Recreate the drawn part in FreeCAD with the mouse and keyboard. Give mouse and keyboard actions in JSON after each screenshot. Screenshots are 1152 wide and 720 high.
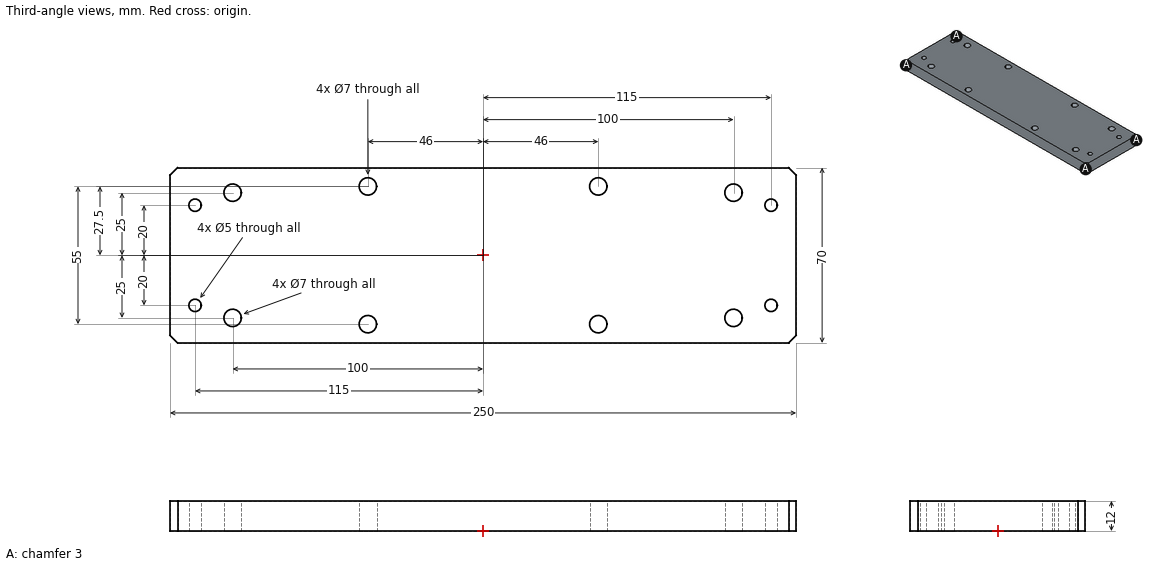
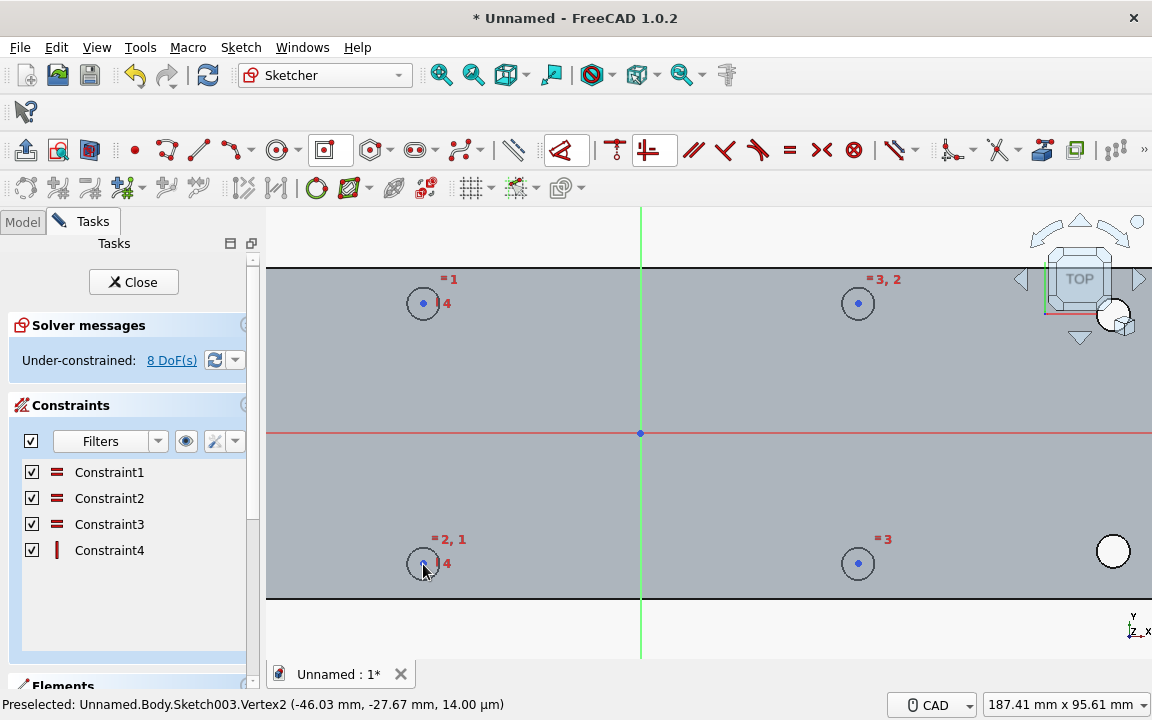
{"action": "left_click", "coordinate": [423, 304]}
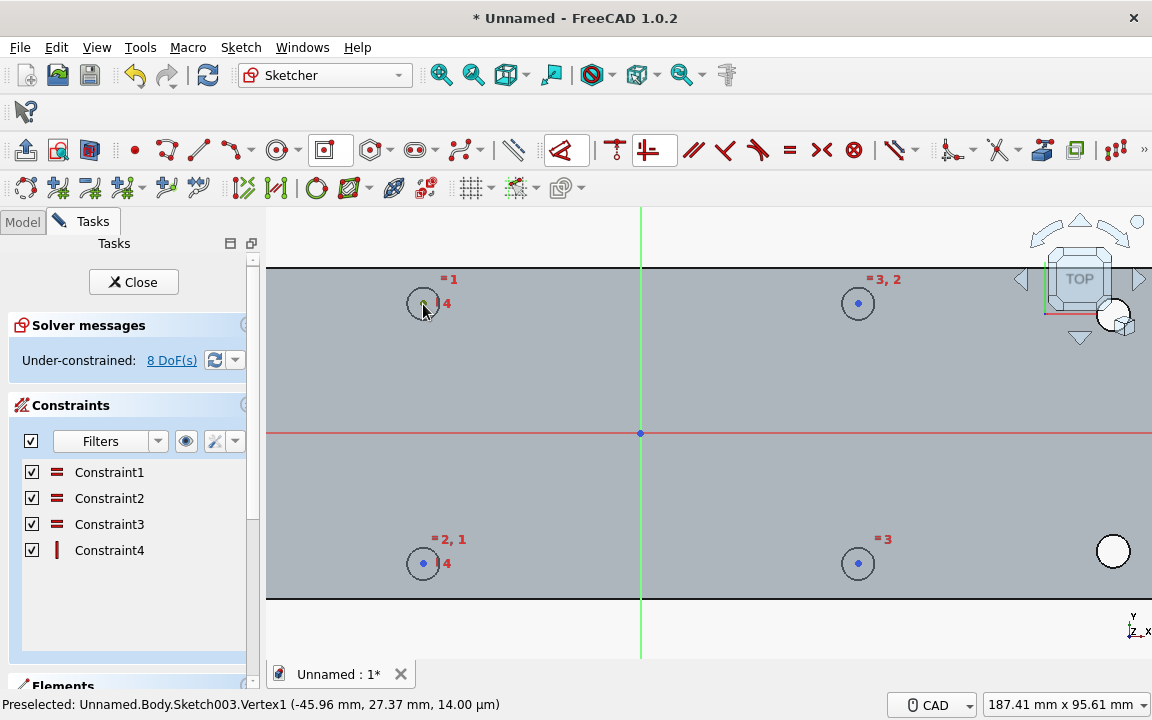
{"action": "left_click", "coordinate": [858, 304]}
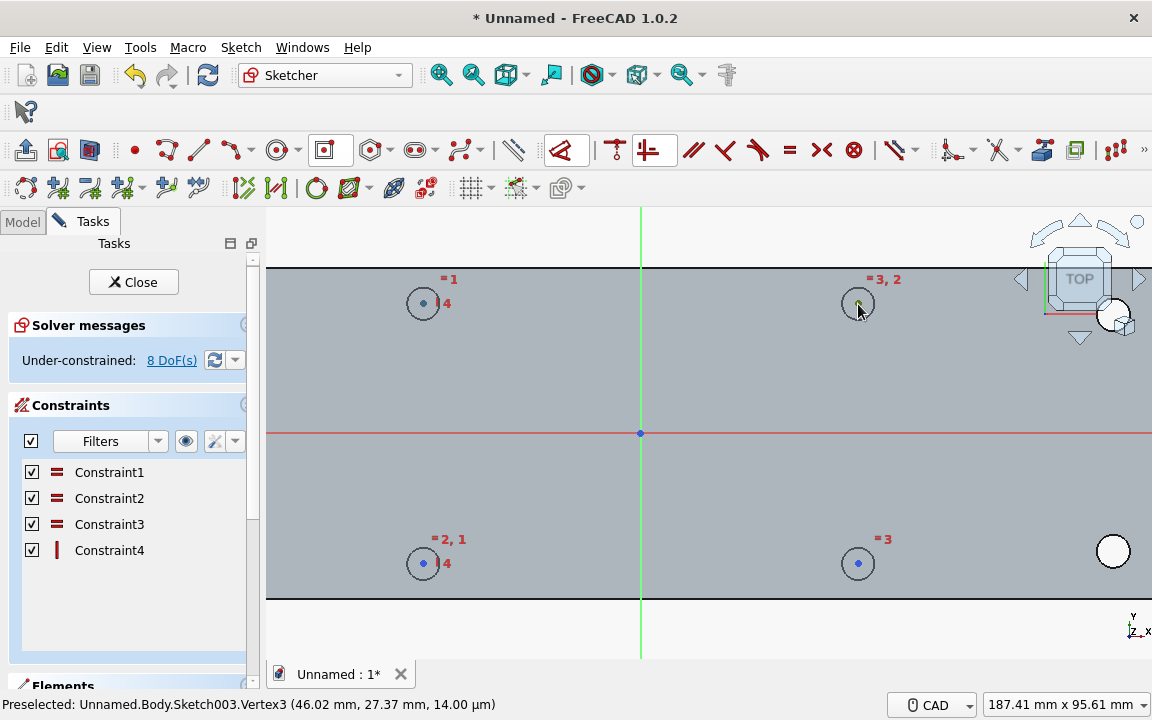
{"action": "left_click", "coordinate": [672, 150]}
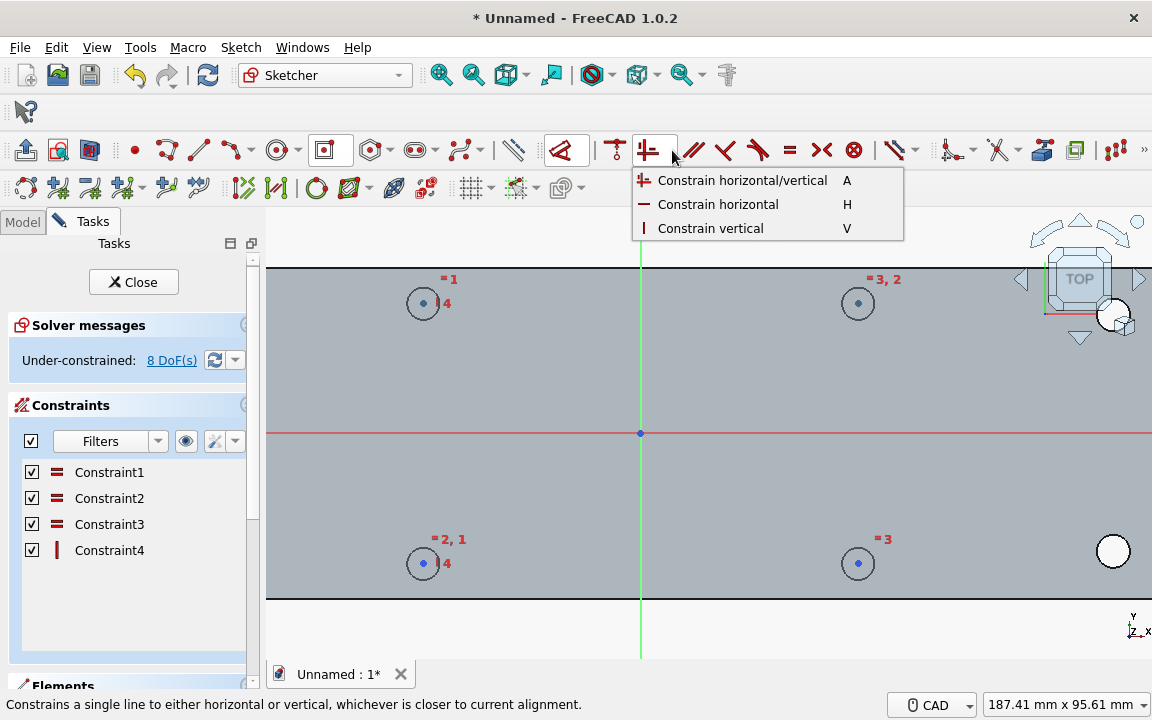
{"action": "left_click", "coordinate": [768, 204]}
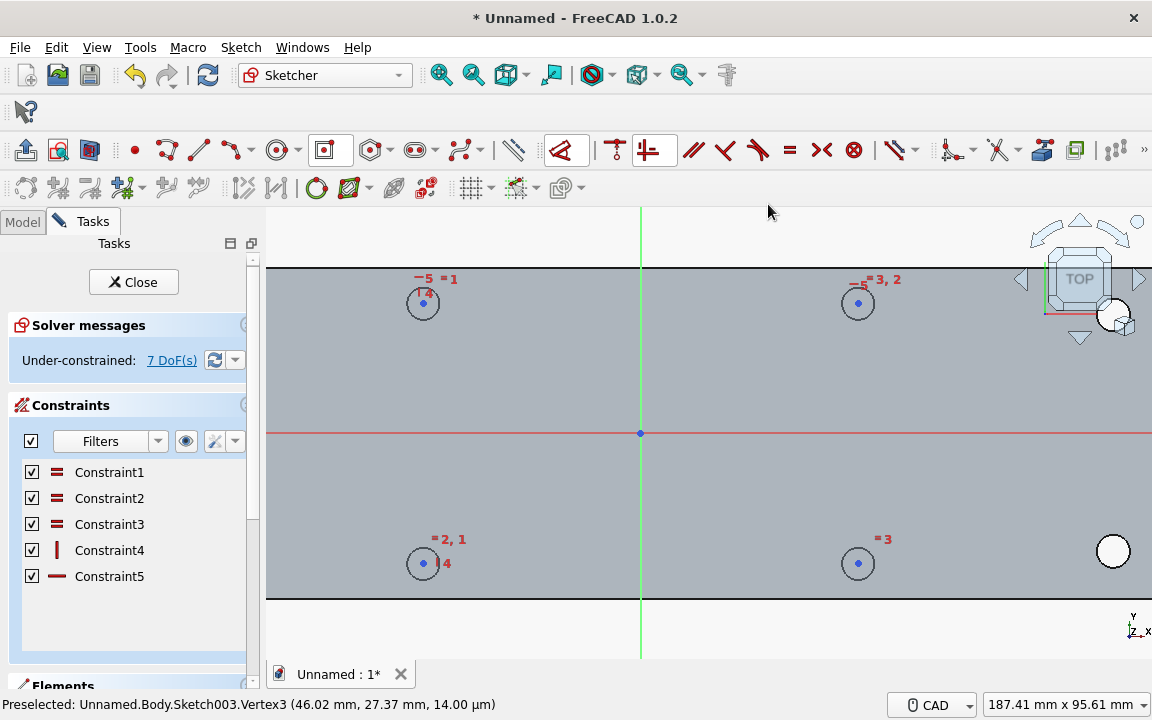
{"action": "left_click", "coordinate": [858, 304]}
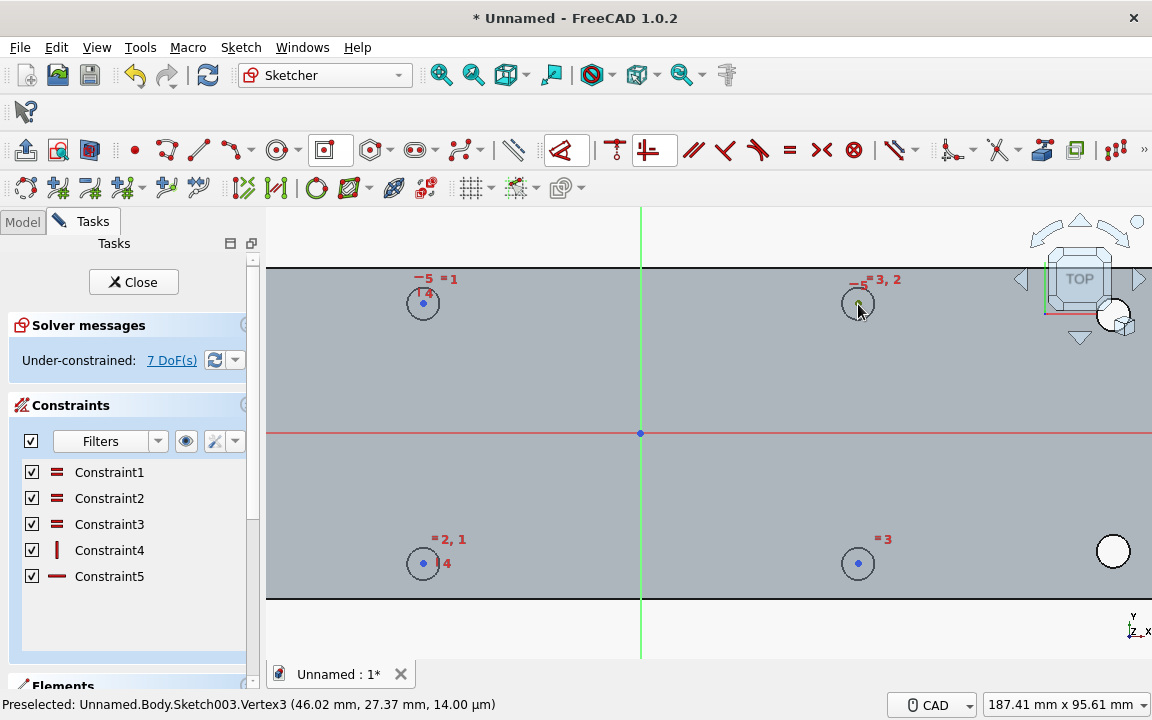
{"action": "left_click", "coordinate": [858, 564]}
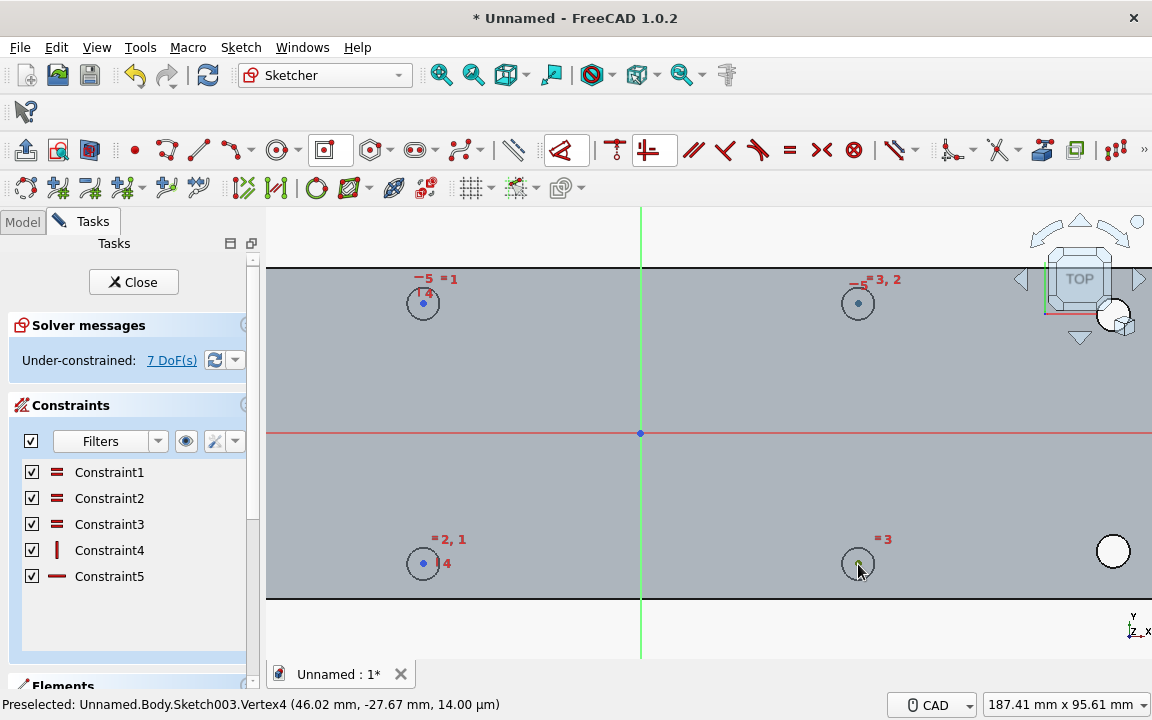
{"action": "key", "text": "v"}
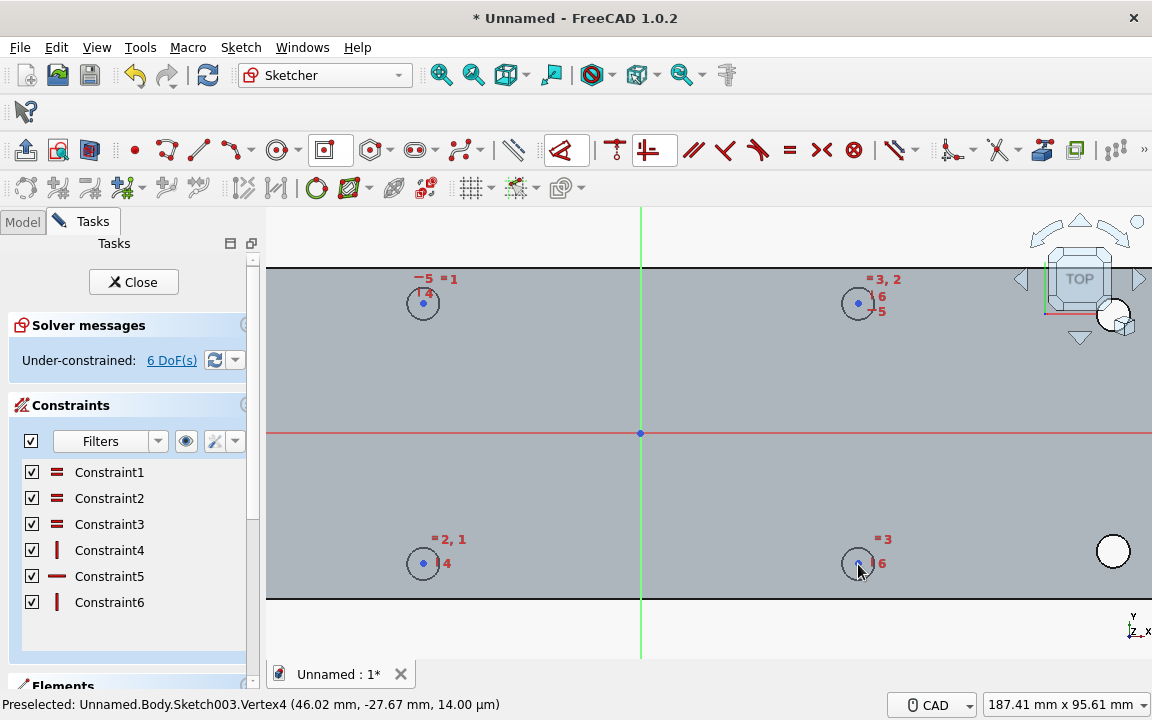
{"action": "left_click", "coordinate": [423, 564]}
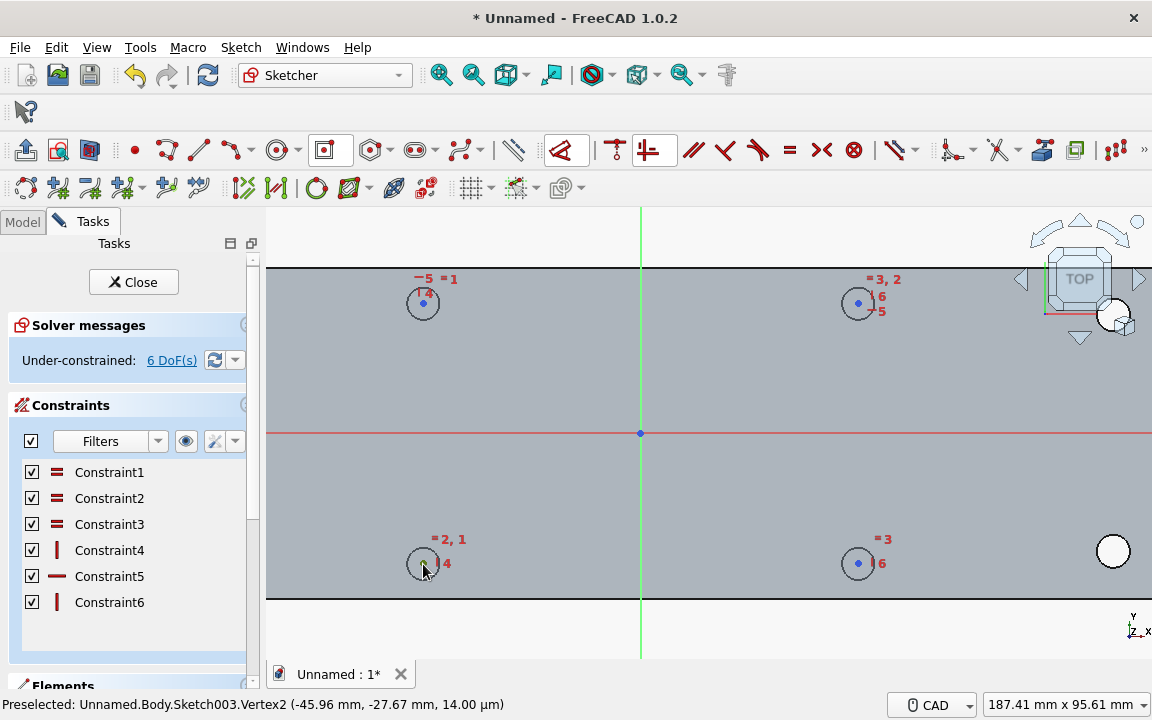
{"action": "left_click", "coordinate": [858, 564]}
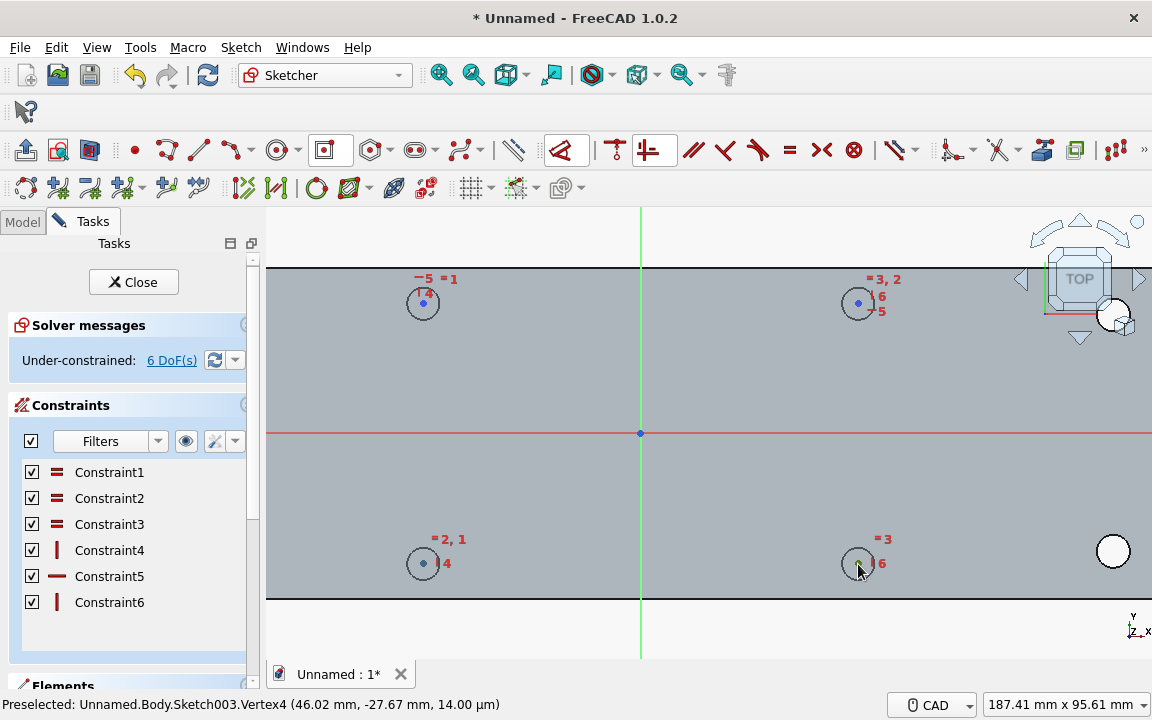
{"action": "left_click", "coordinate": [672, 150]}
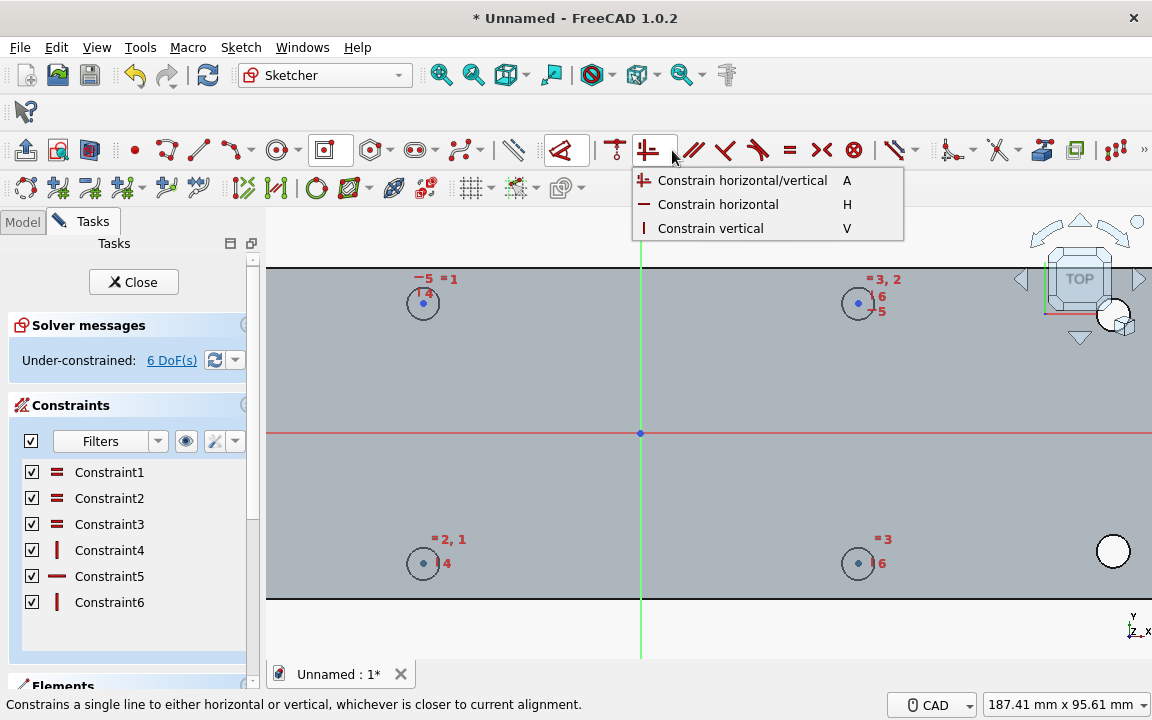
{"action": "left_click", "coordinate": [768, 204]}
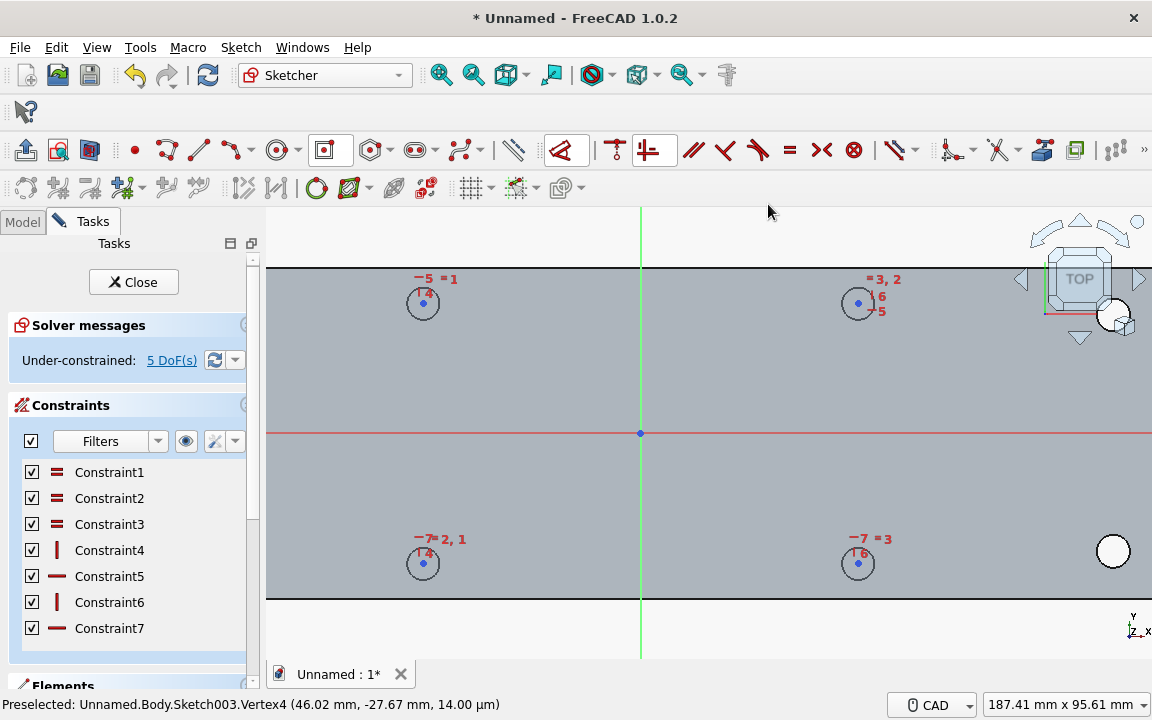
{"action": "left_click", "coordinate": [435, 292]}